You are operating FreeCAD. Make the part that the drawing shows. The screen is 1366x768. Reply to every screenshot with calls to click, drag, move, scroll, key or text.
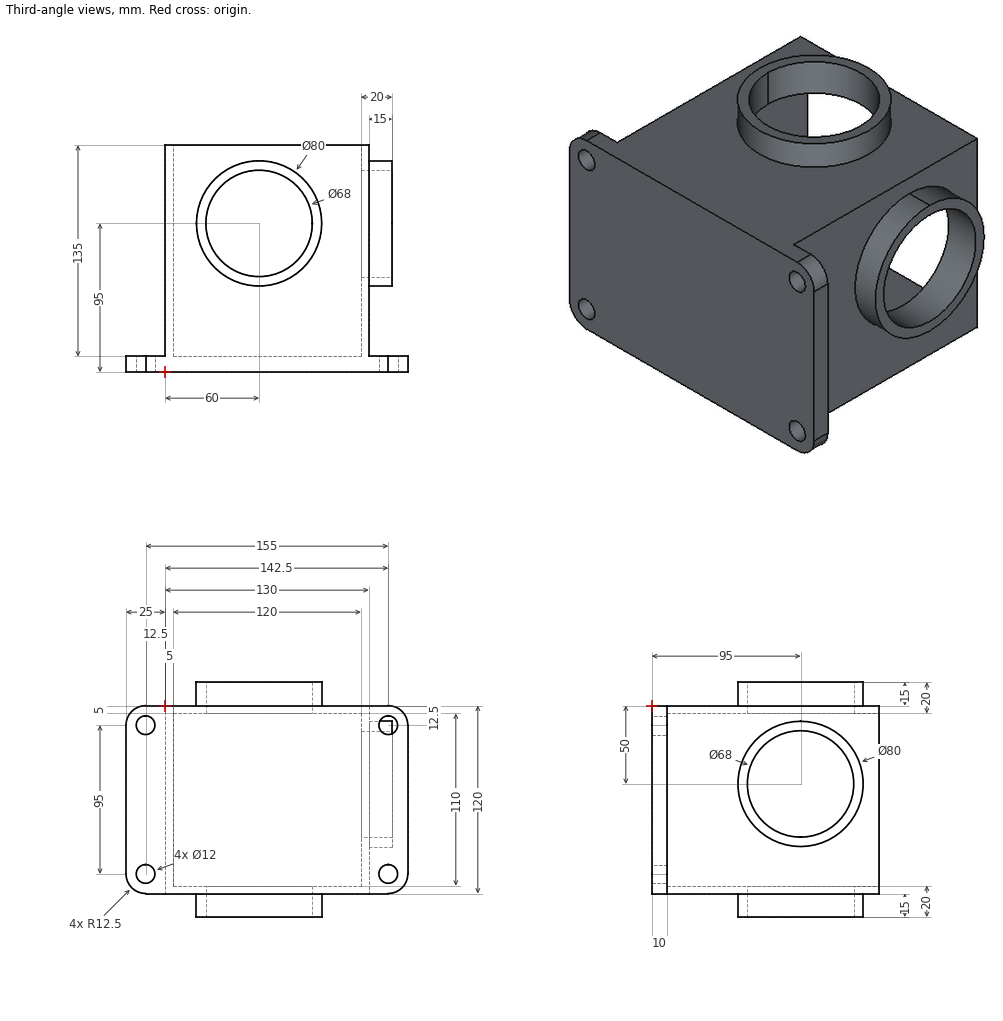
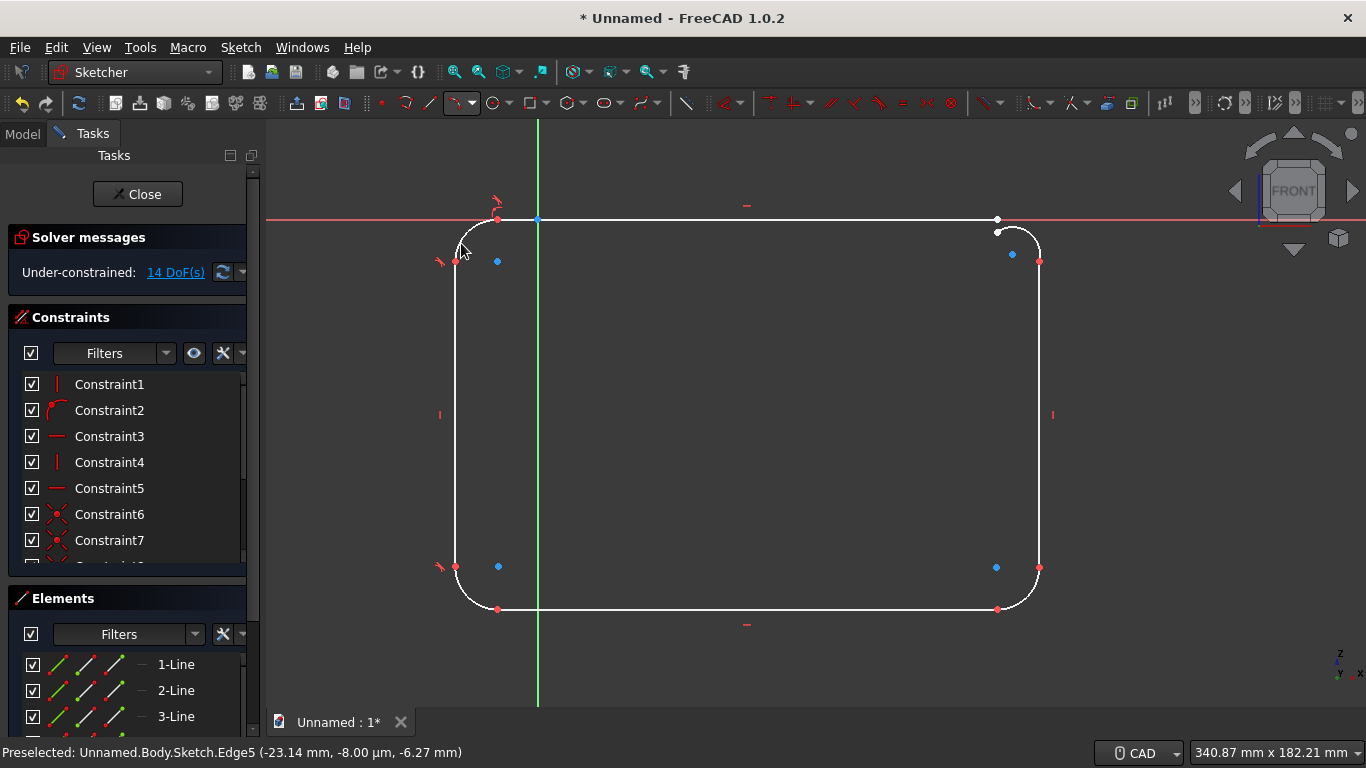
click(648, 220)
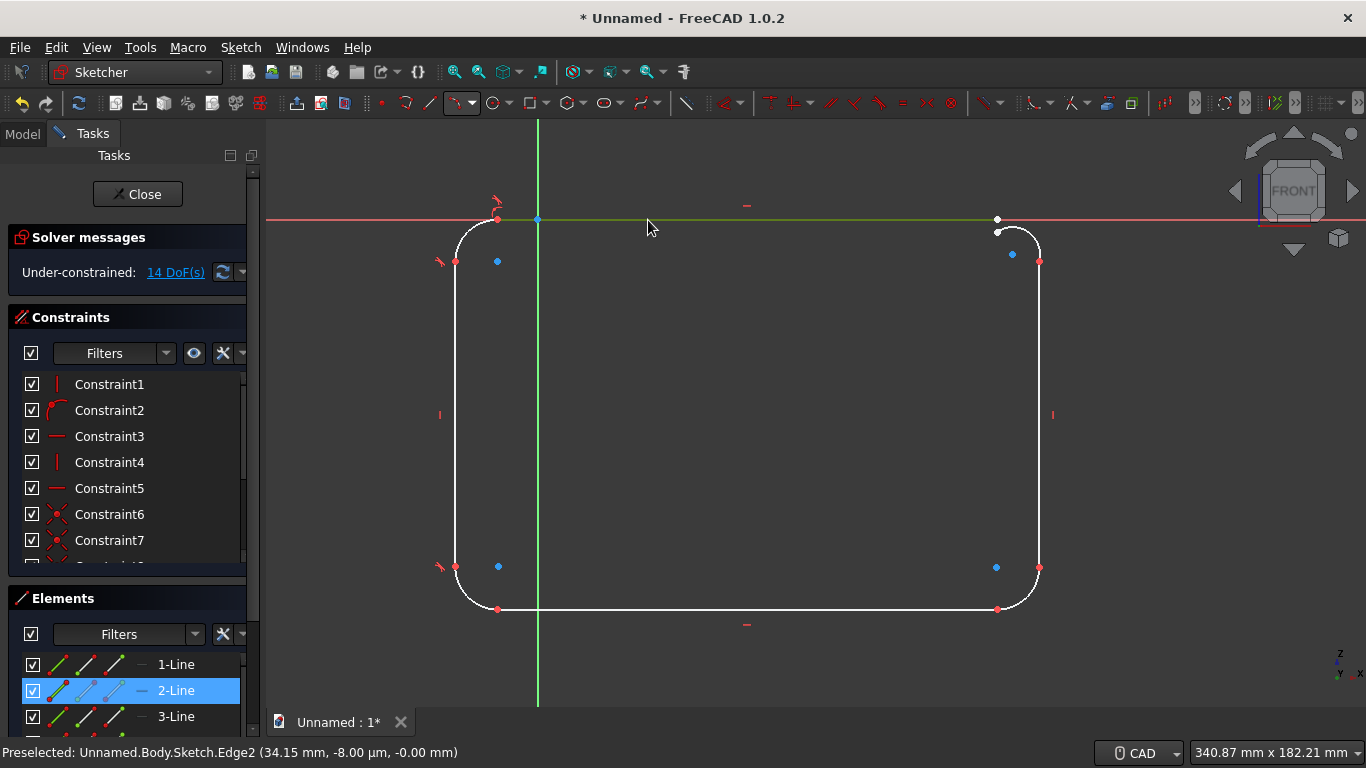
click(1037, 242)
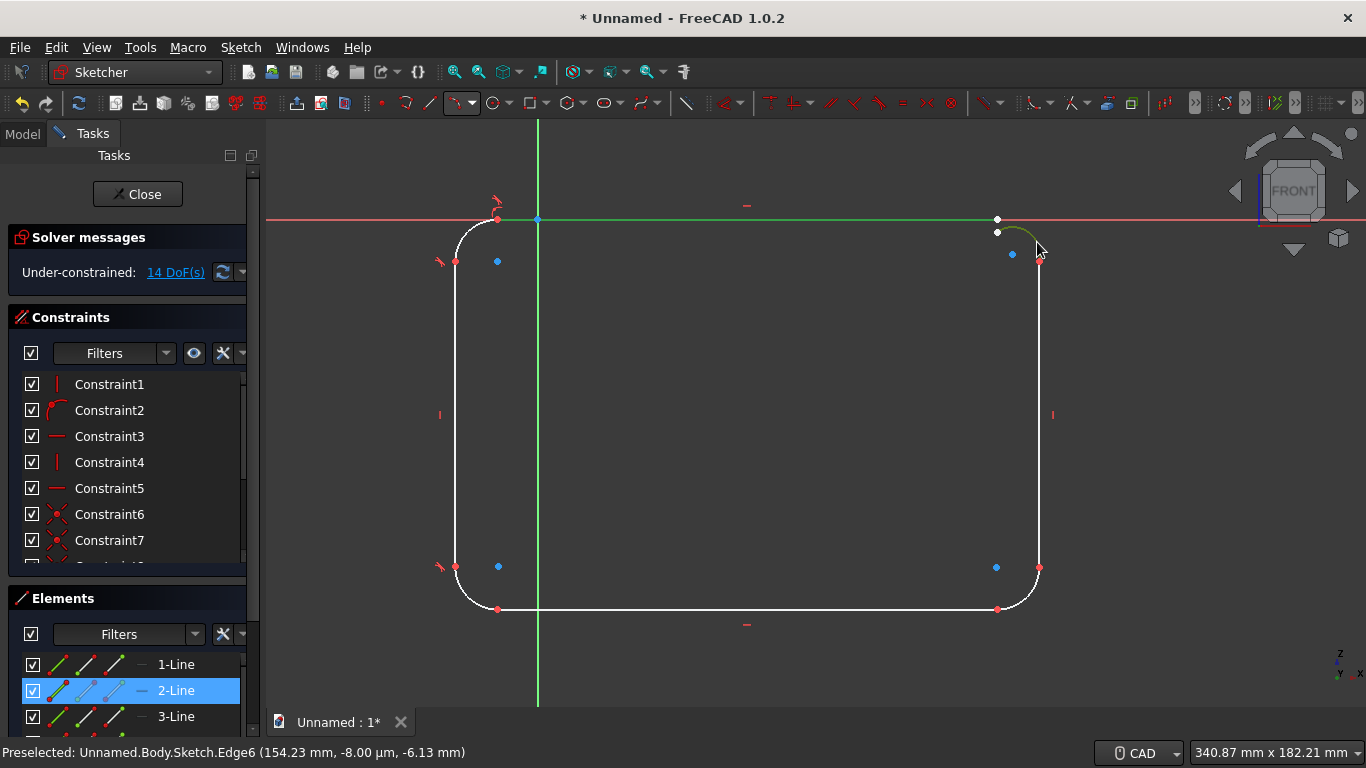
click(880, 104)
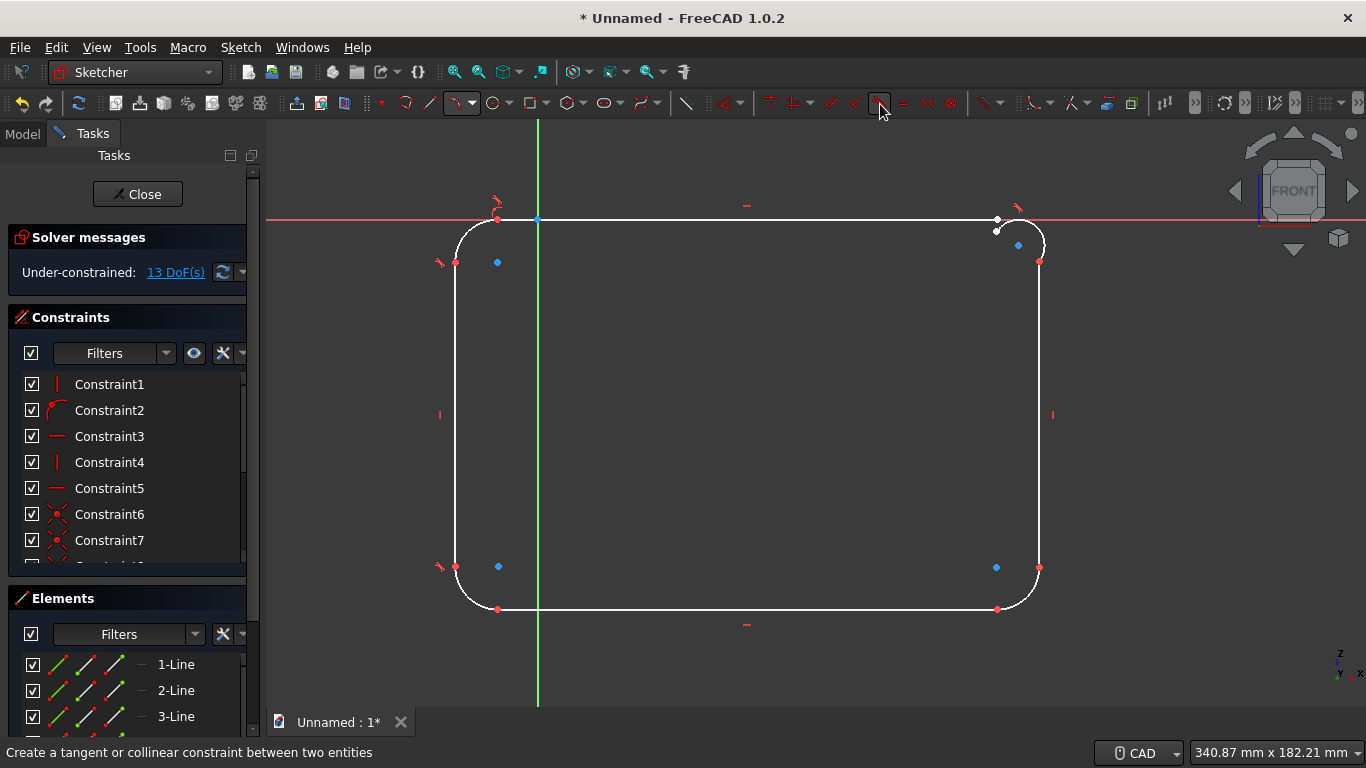
click(1039, 353)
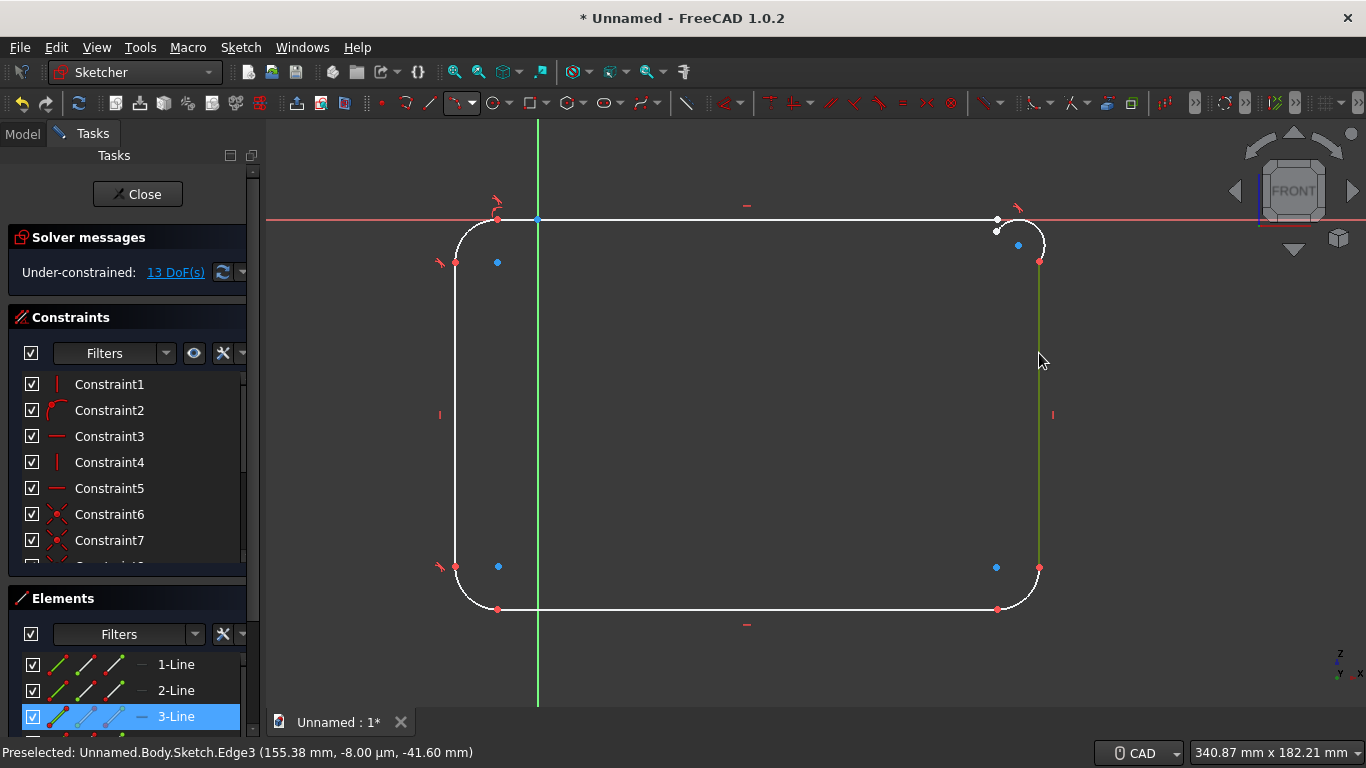
click(1043, 237)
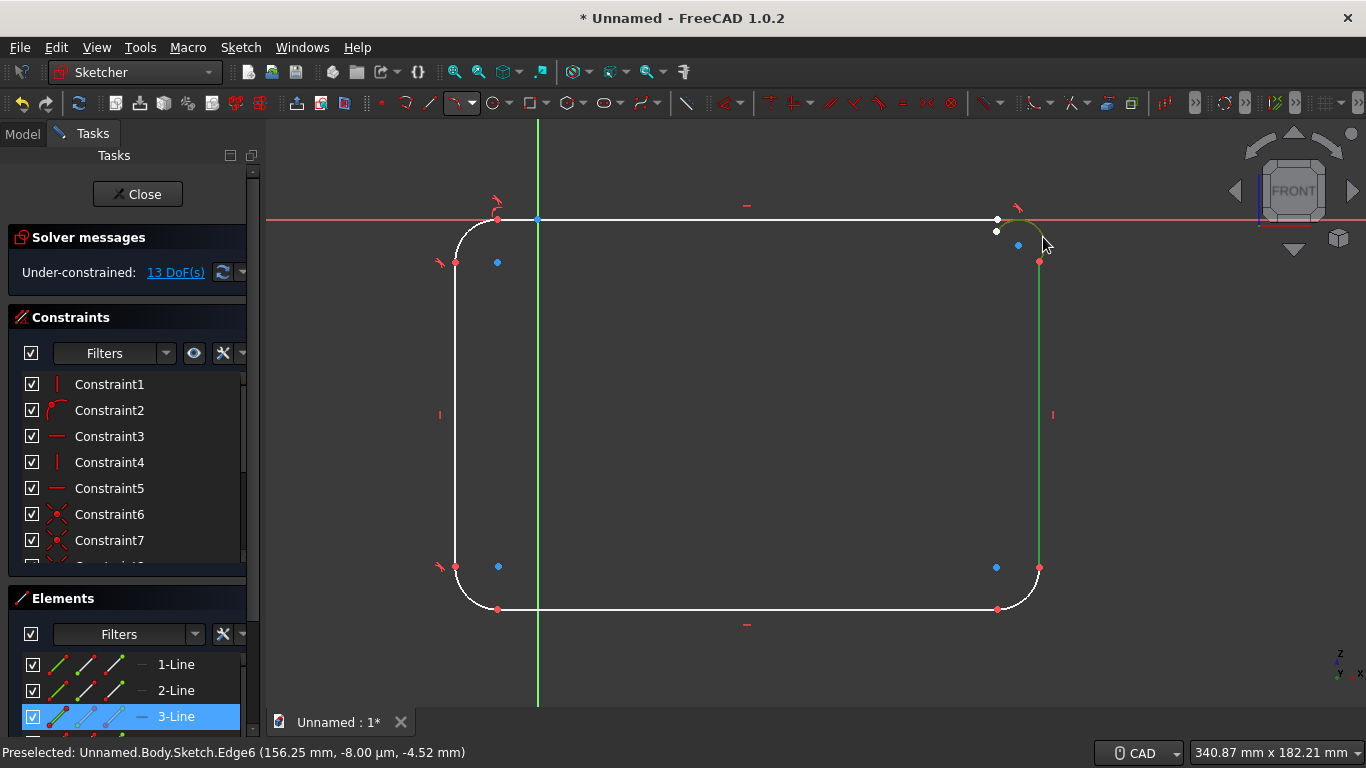
click(880, 104)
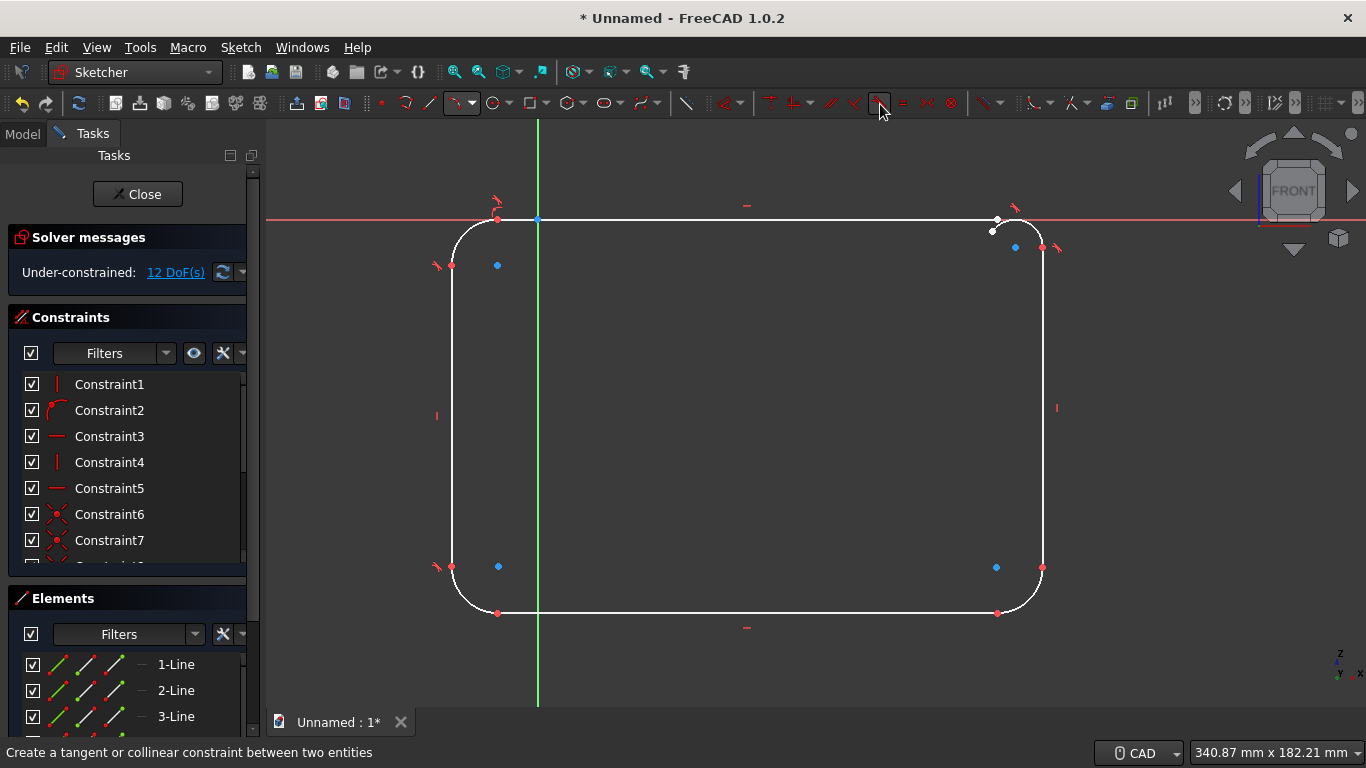
click(1043, 343)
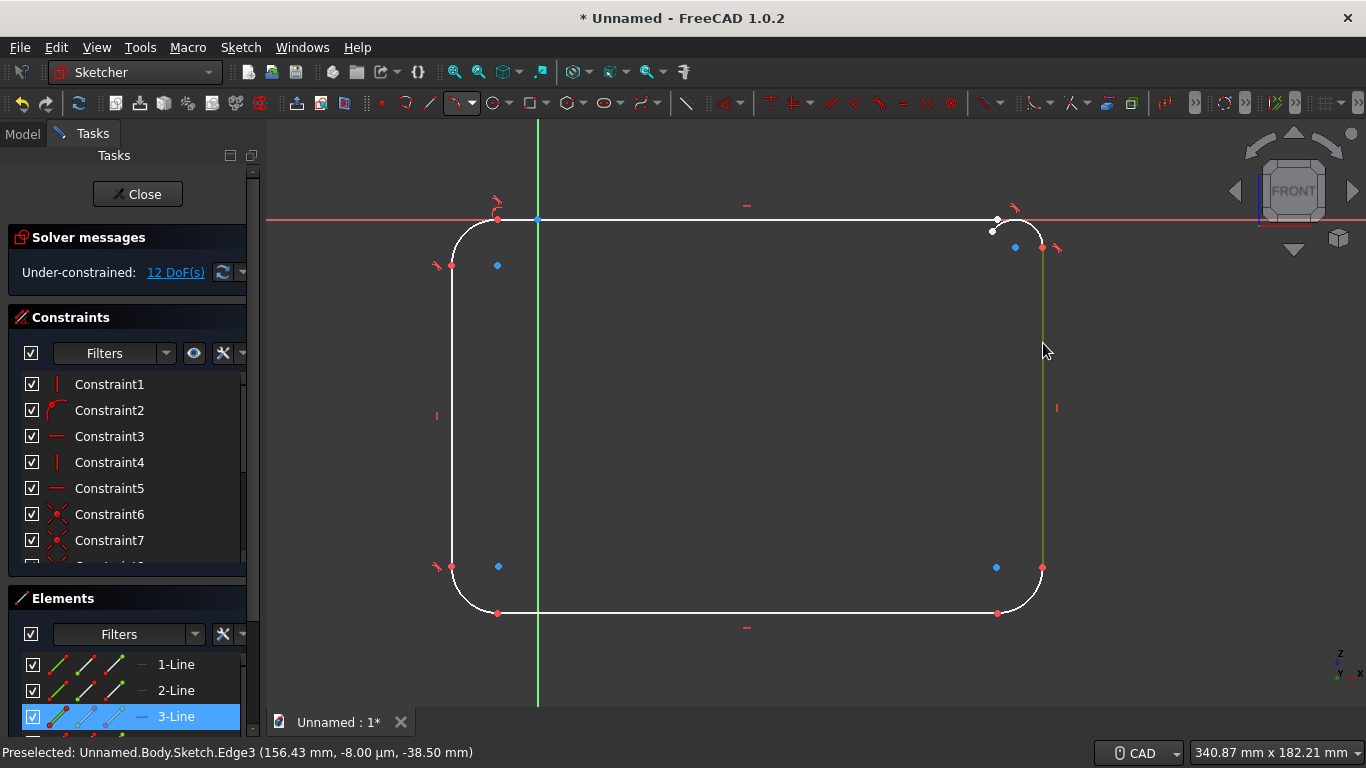
click(1018, 608)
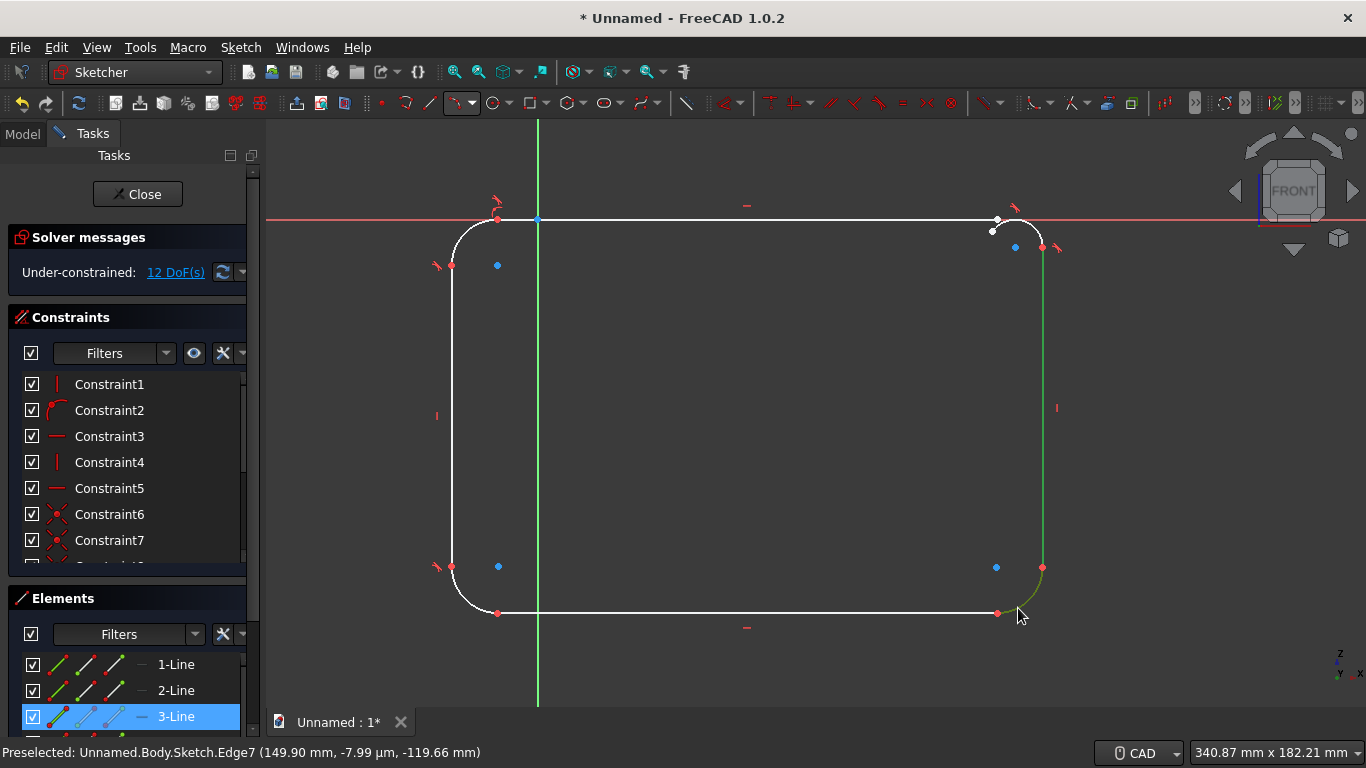
click(880, 104)